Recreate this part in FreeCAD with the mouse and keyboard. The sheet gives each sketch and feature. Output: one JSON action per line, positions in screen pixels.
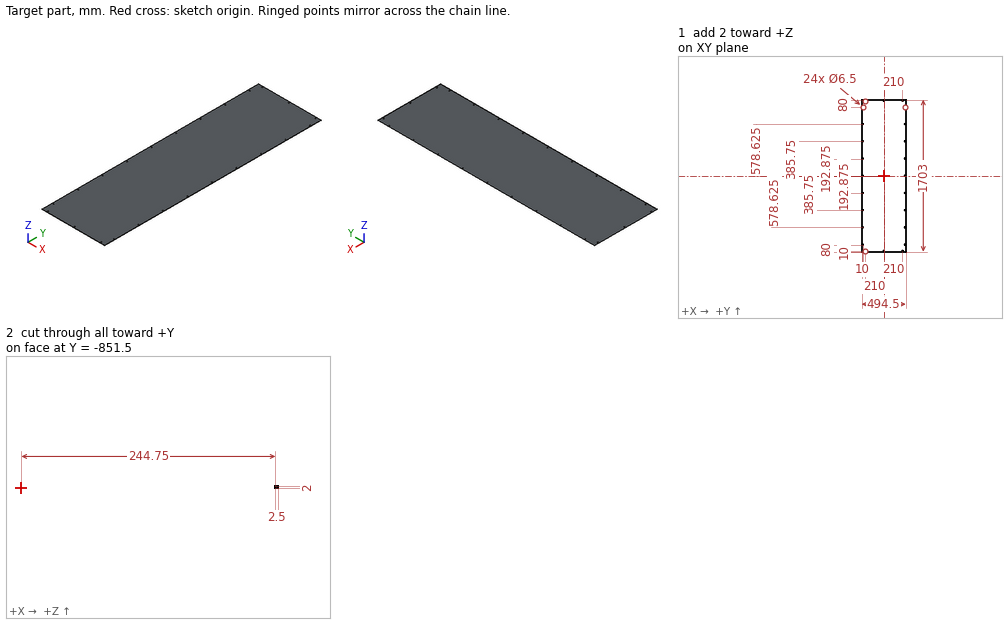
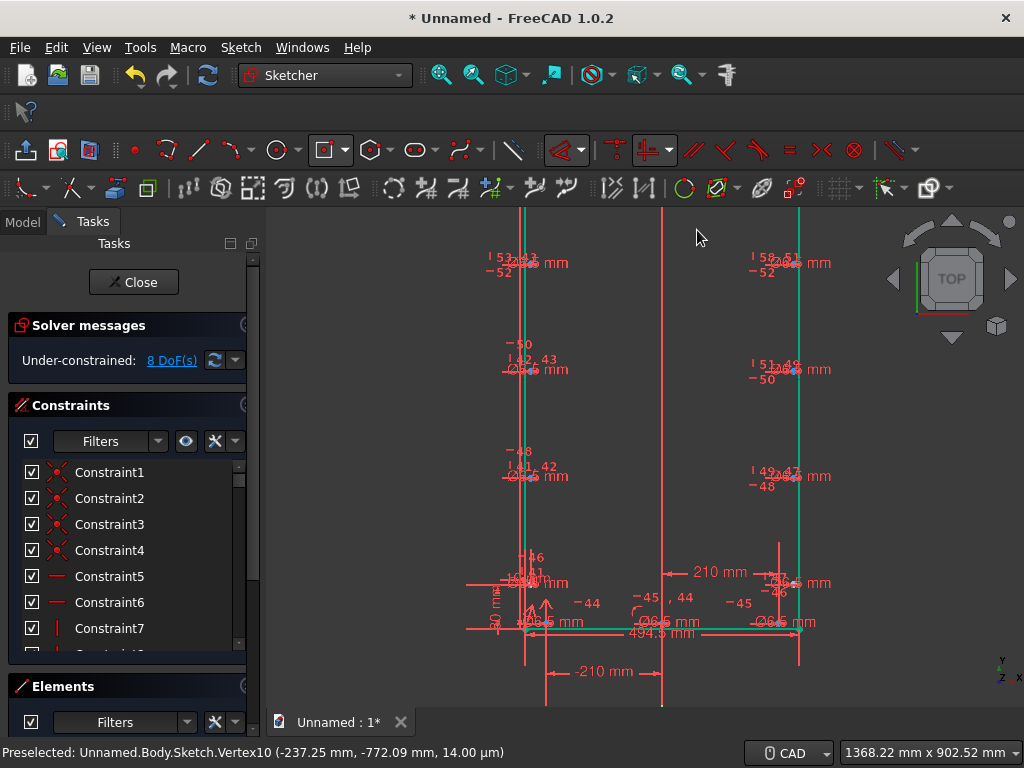
{"action": "scroll", "coordinate": [525, 629], "scroll_direction": "up", "scroll_amount": 10}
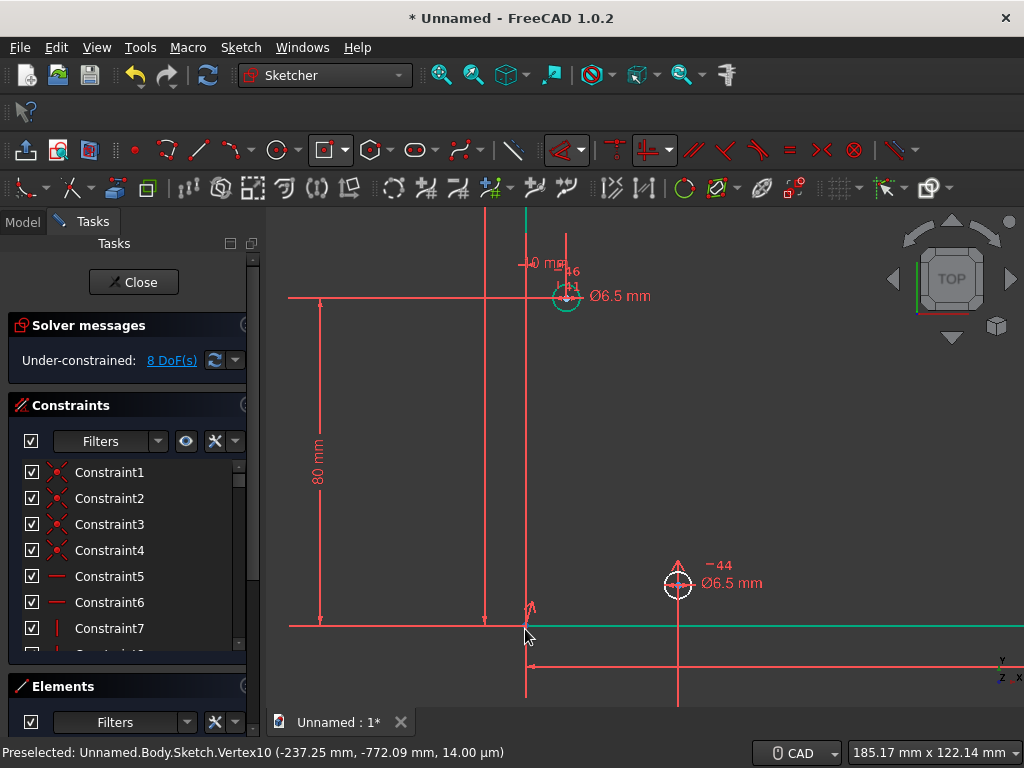
{"action": "left_click", "coordinate": [526, 626]}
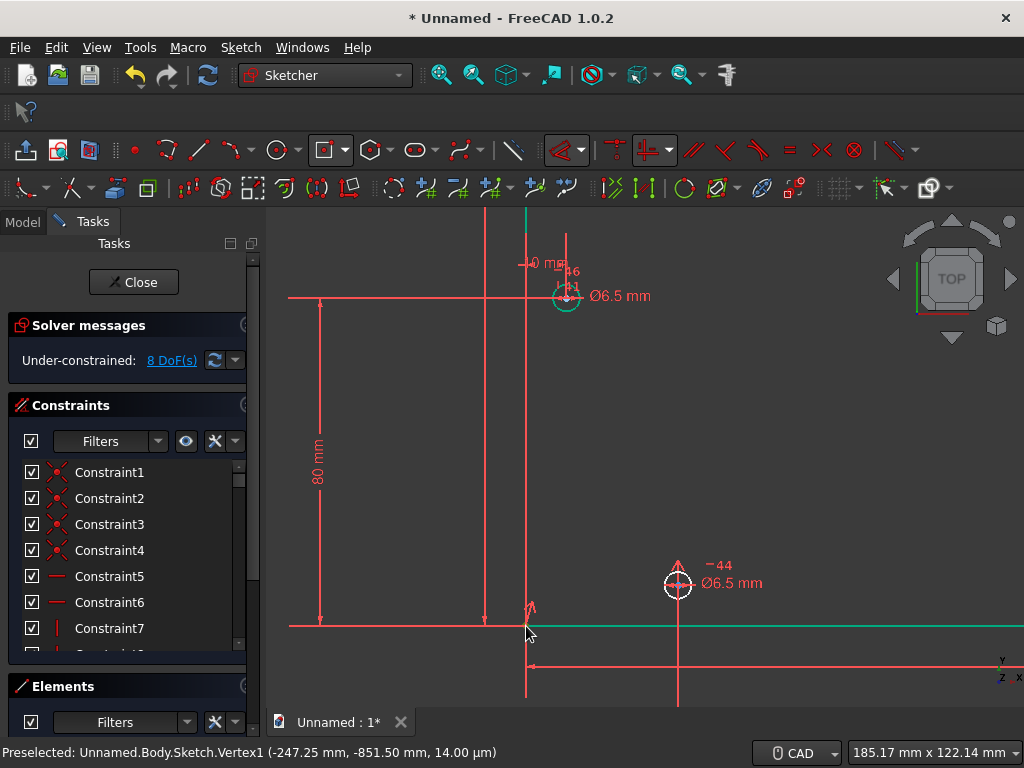
{"action": "left_click", "coordinate": [678, 585]}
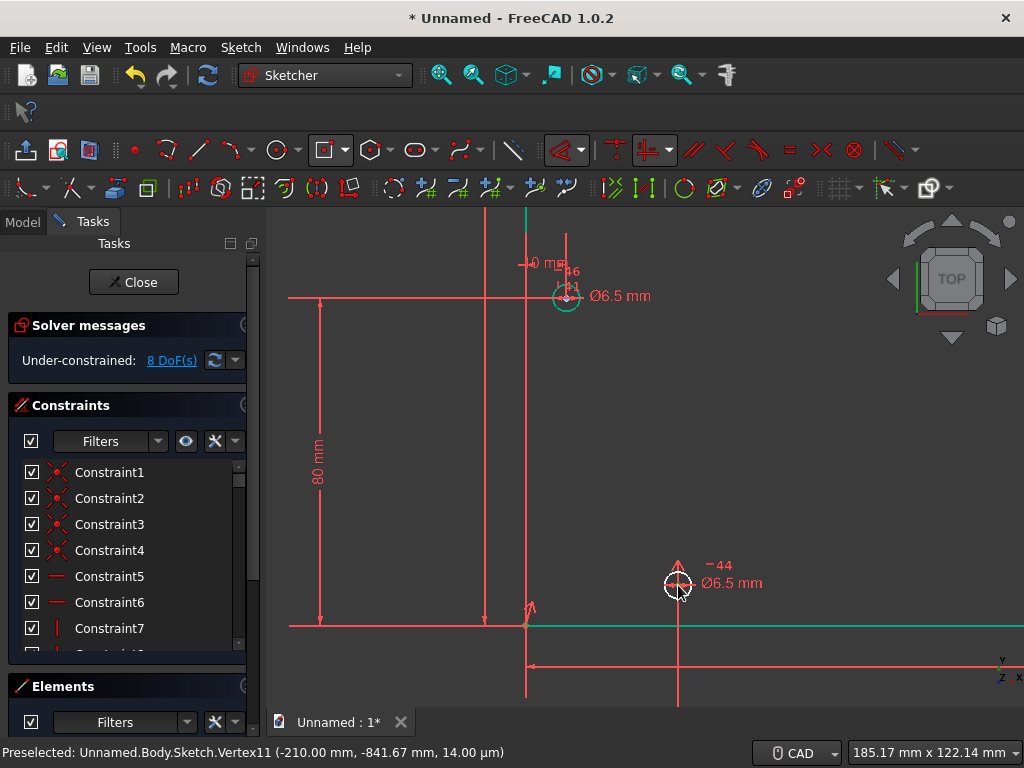
{"action": "key", "text": "i"}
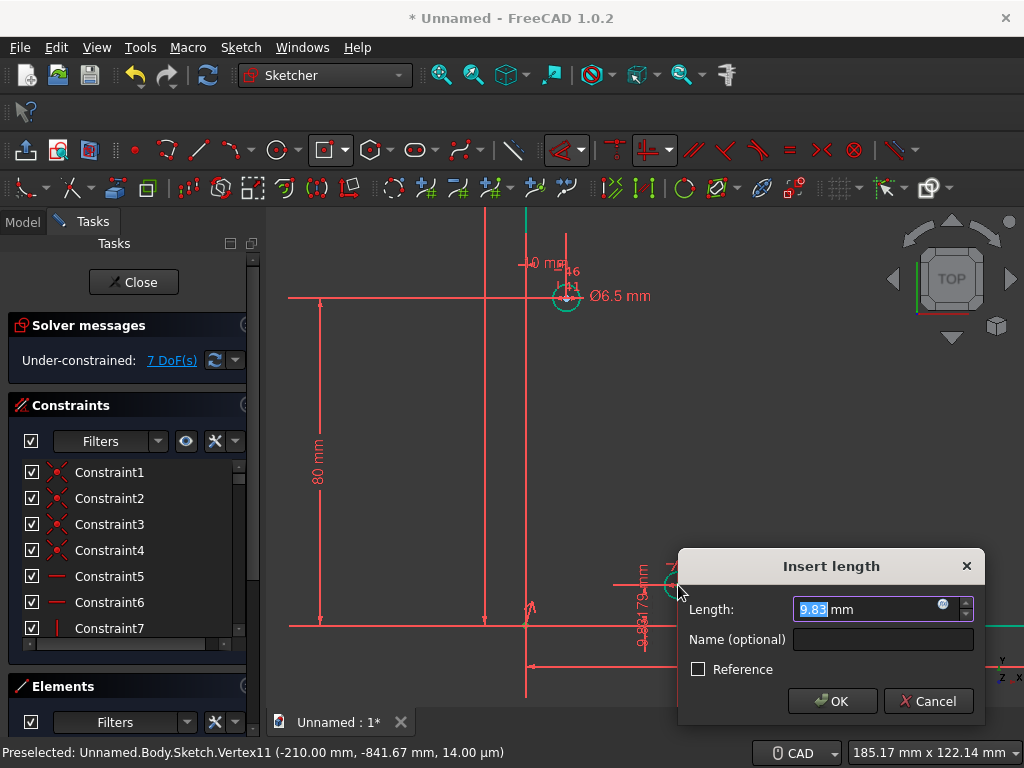
{"action": "type", "text": "10"}
{"action": "key", "text": "Return"}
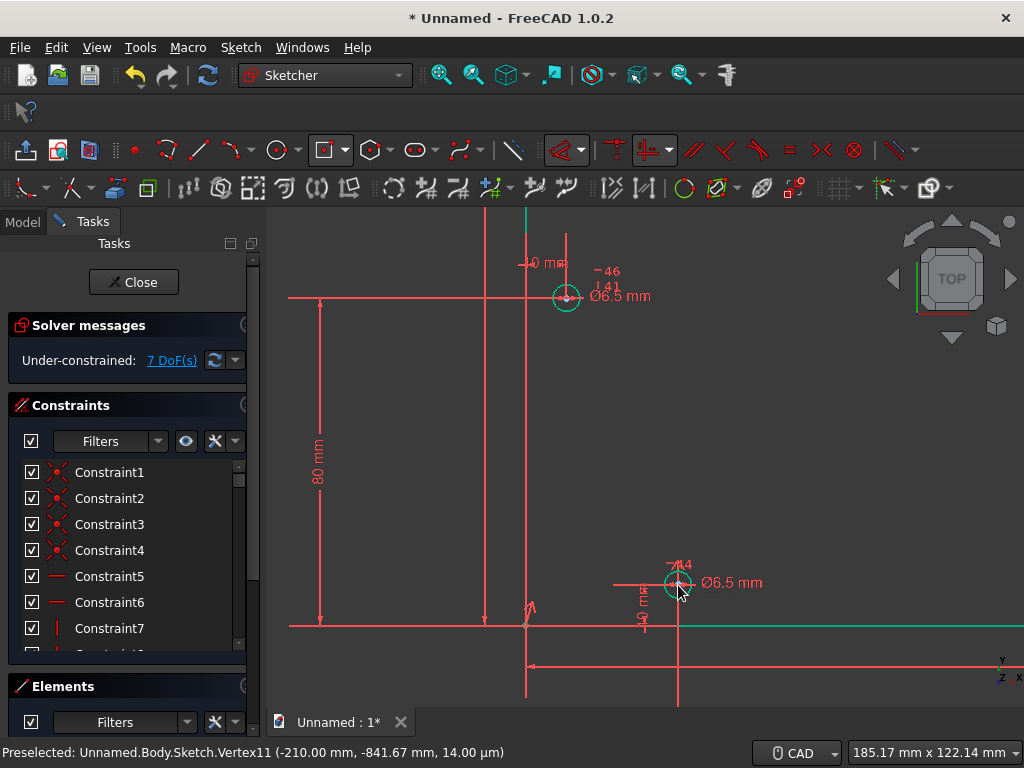
{"action": "scroll", "coordinate": [526, 631], "scroll_direction": "down", "scroll_amount": 15}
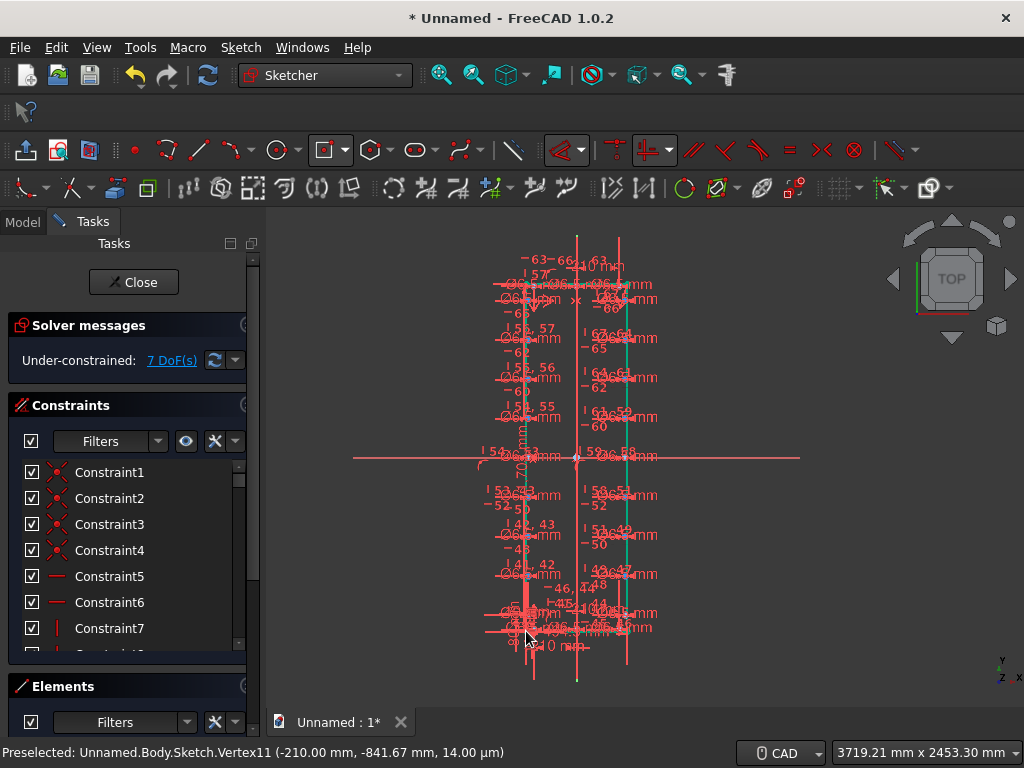
{"action": "scroll", "coordinate": [526, 284], "scroll_direction": "up", "scroll_amount": 5}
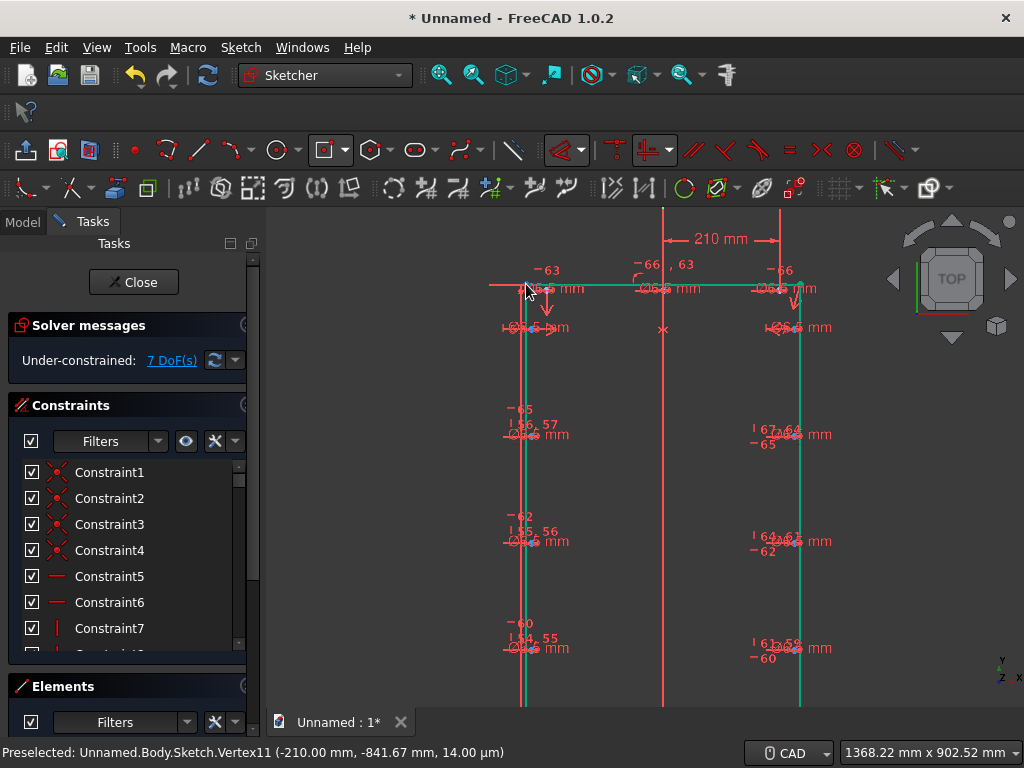
{"action": "left_click", "coordinate": [526, 285]}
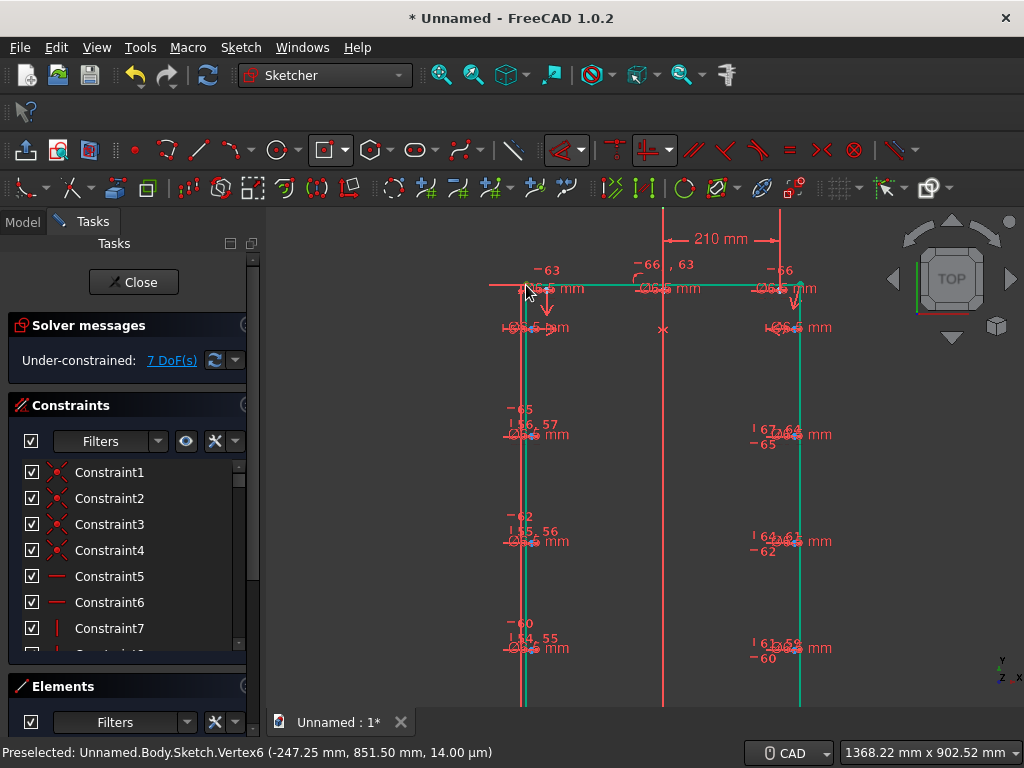
{"action": "left_click", "coordinate": [532, 329]}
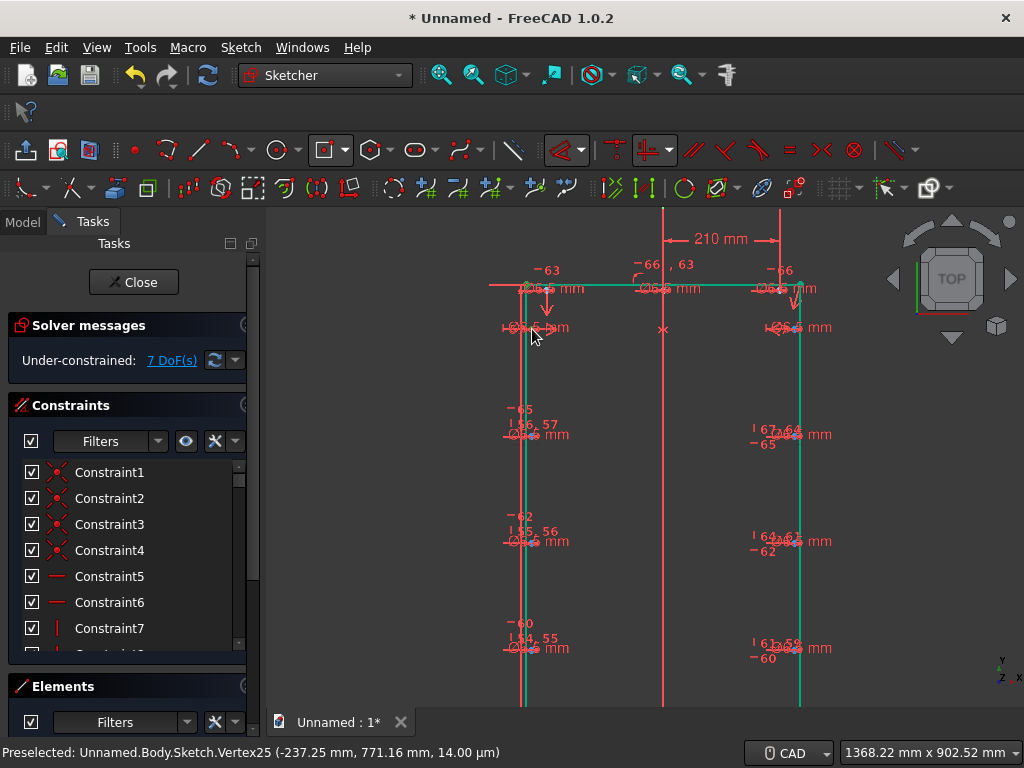
{"action": "key", "text": "i"}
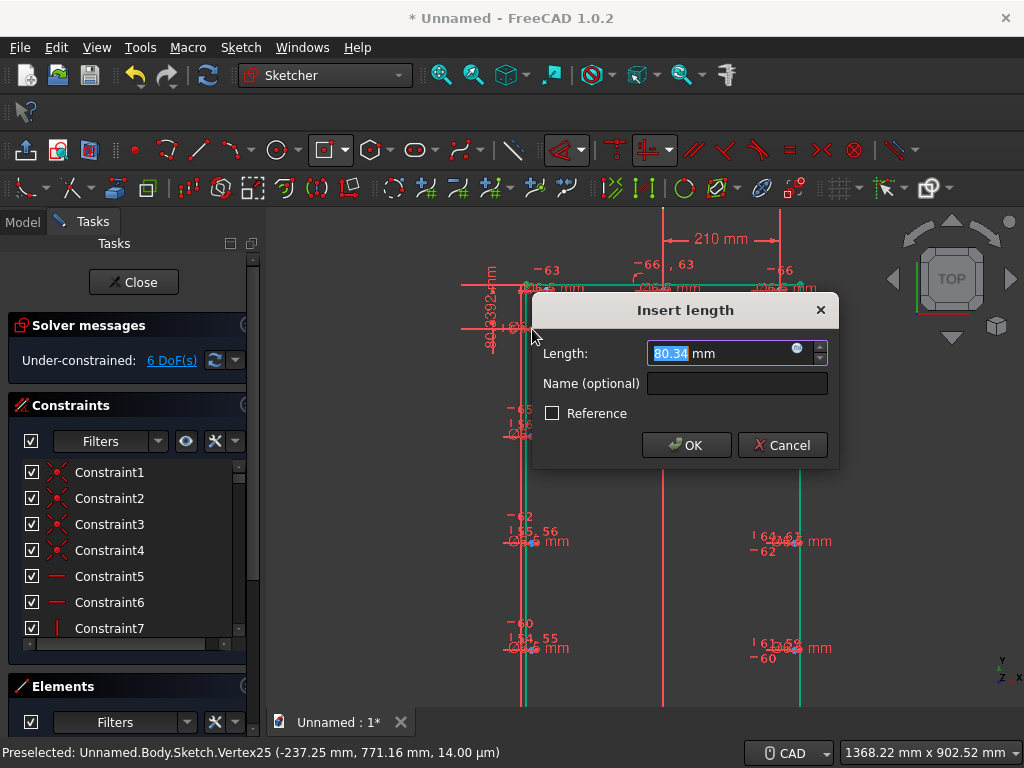
{"action": "type", "text": "80"}
{"action": "key", "text": "Return"}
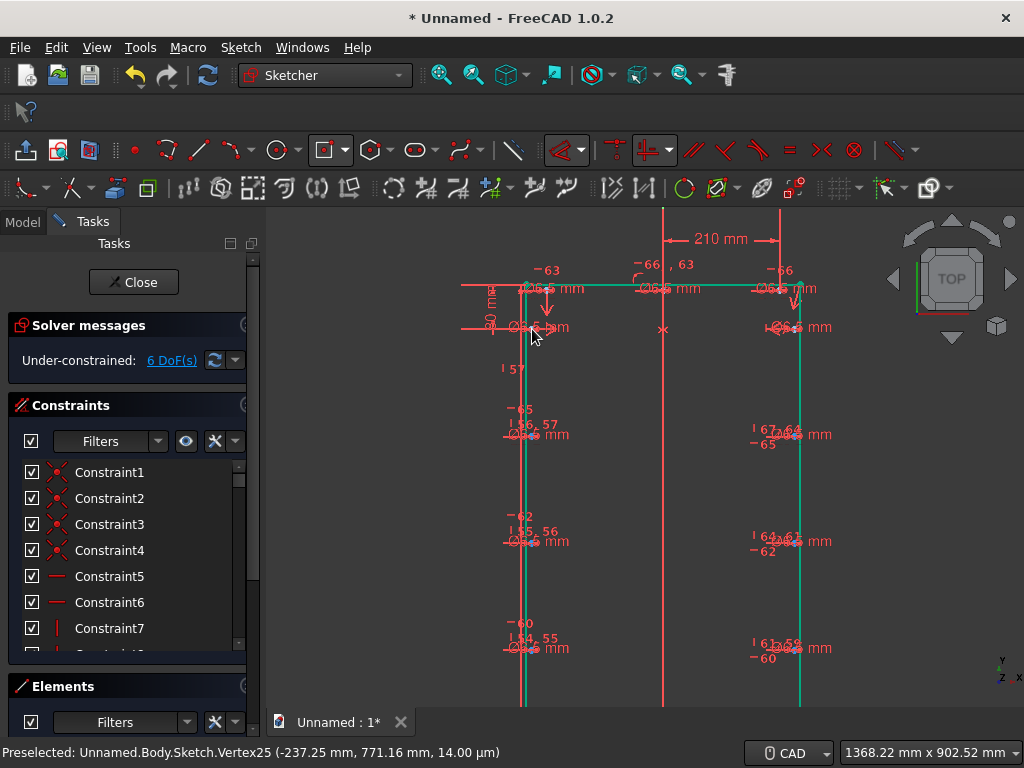
{"action": "scroll", "coordinate": [539, 328], "scroll_direction": "down", "scroll_amount": 6}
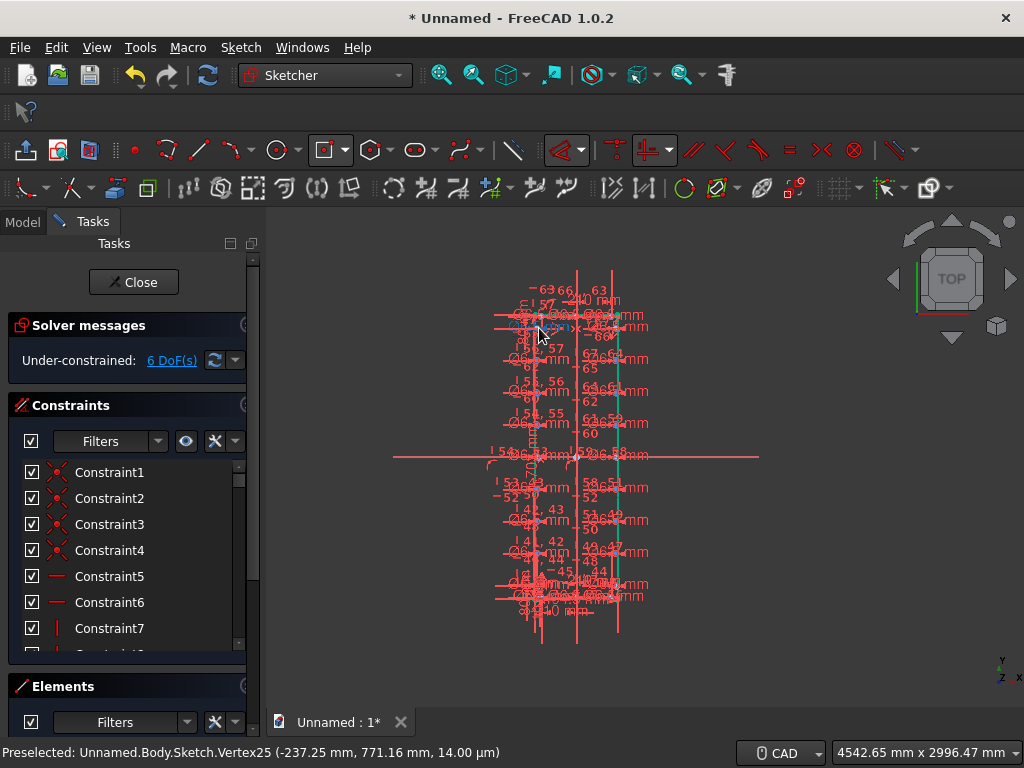
{"action": "left_click", "coordinate": [537, 522]}